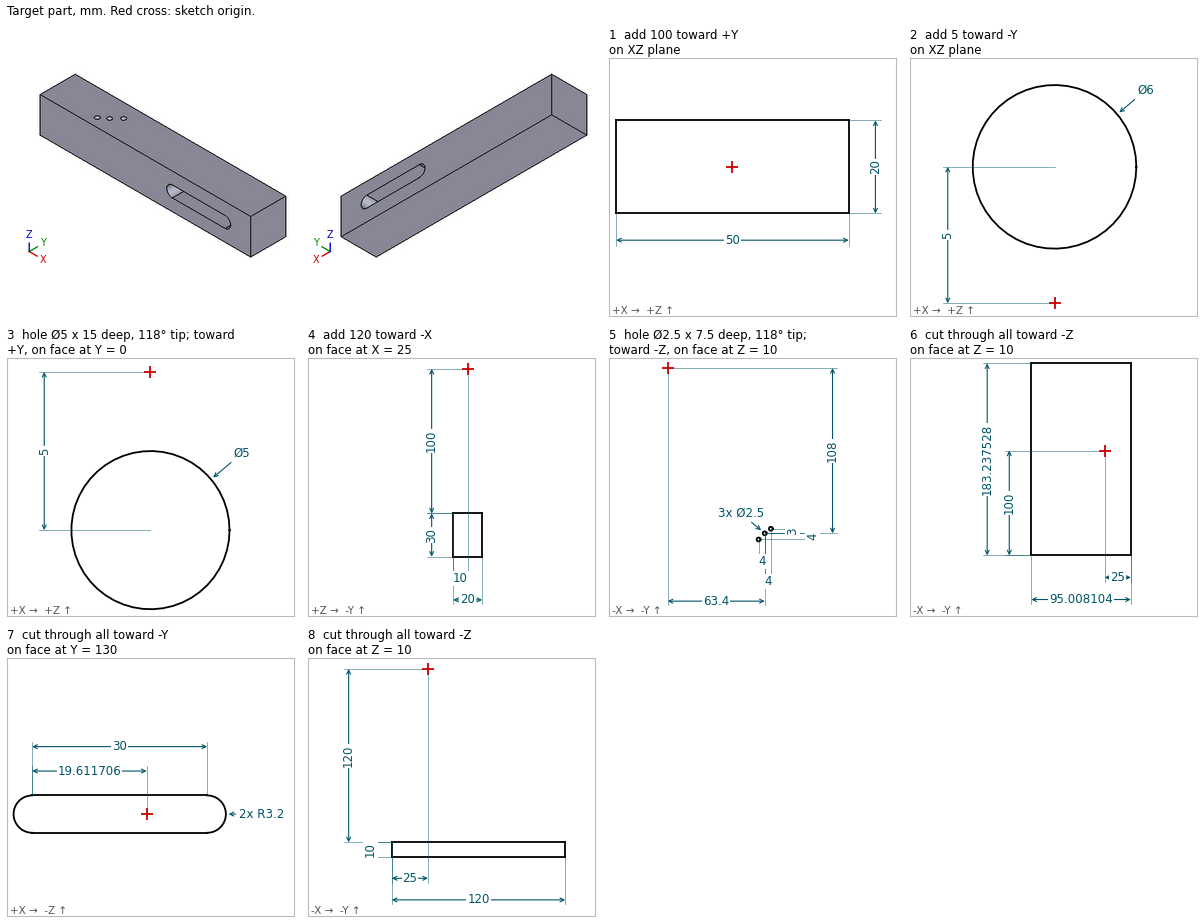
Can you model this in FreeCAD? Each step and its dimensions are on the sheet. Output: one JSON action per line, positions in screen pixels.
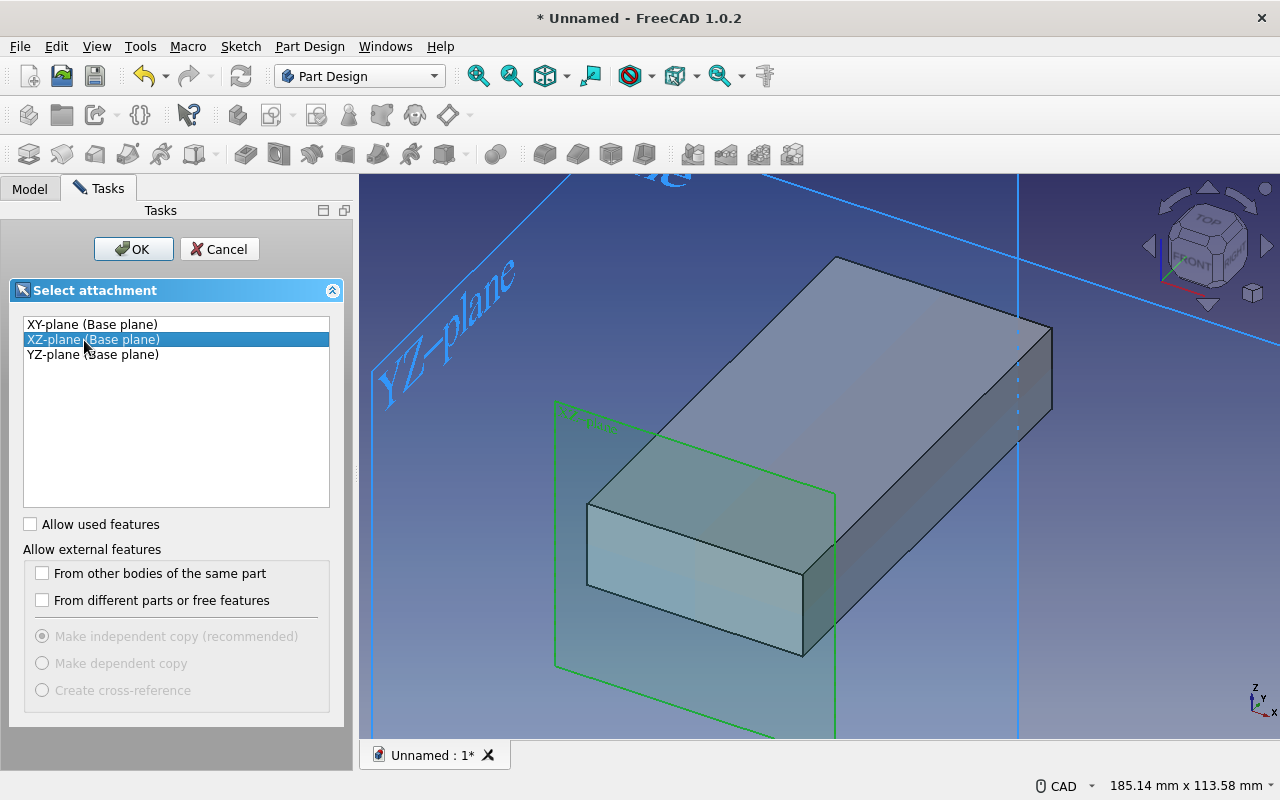
{"action": "left_click", "coordinate": [134, 249]}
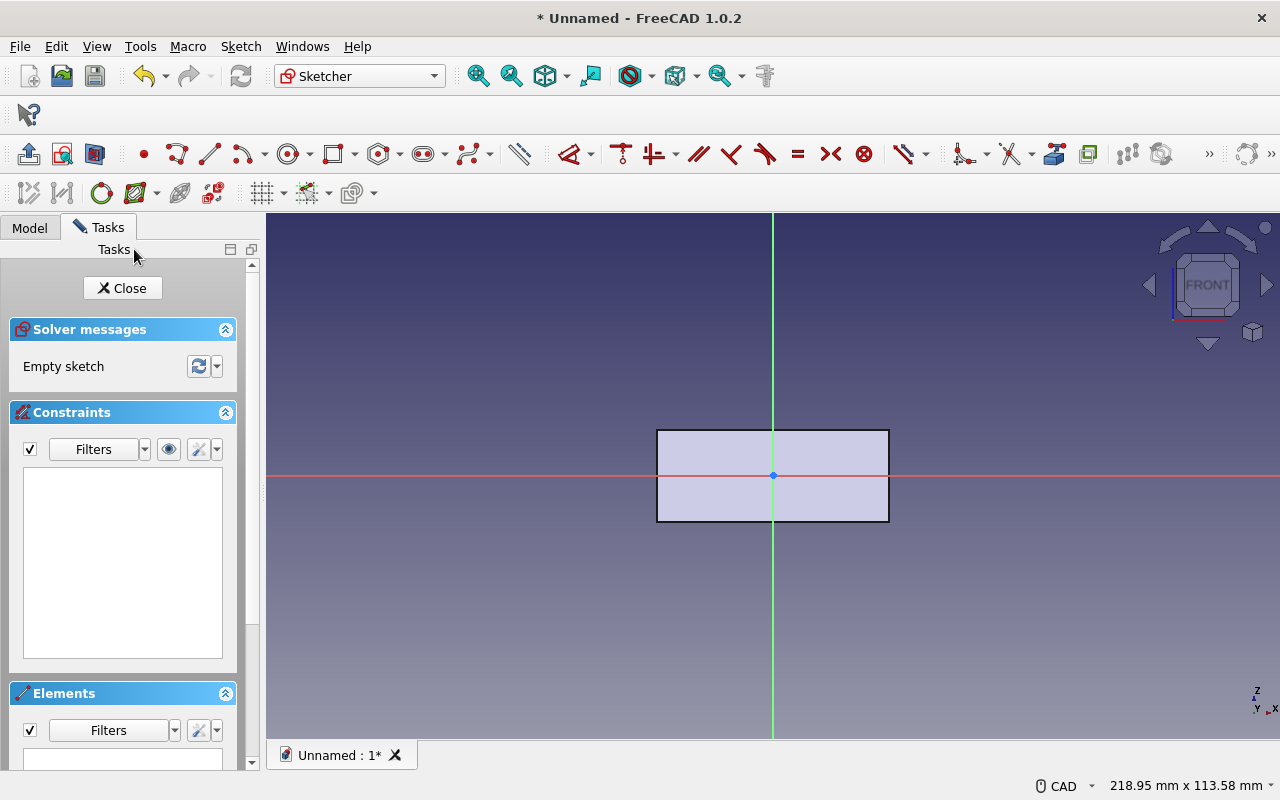
{"action": "scroll", "coordinate": [782, 455], "scroll_direction": "up", "scroll_amount": 11}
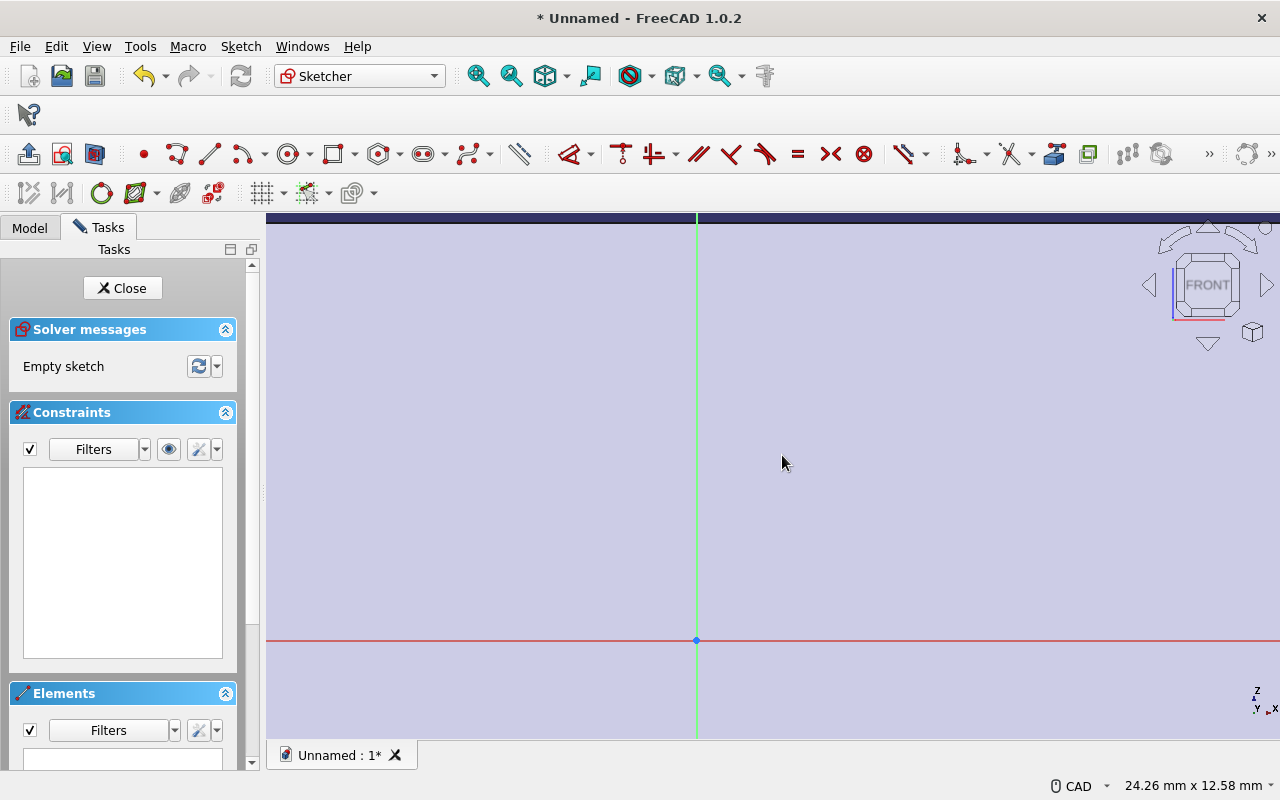
{"action": "left_click", "coordinate": [288, 154]}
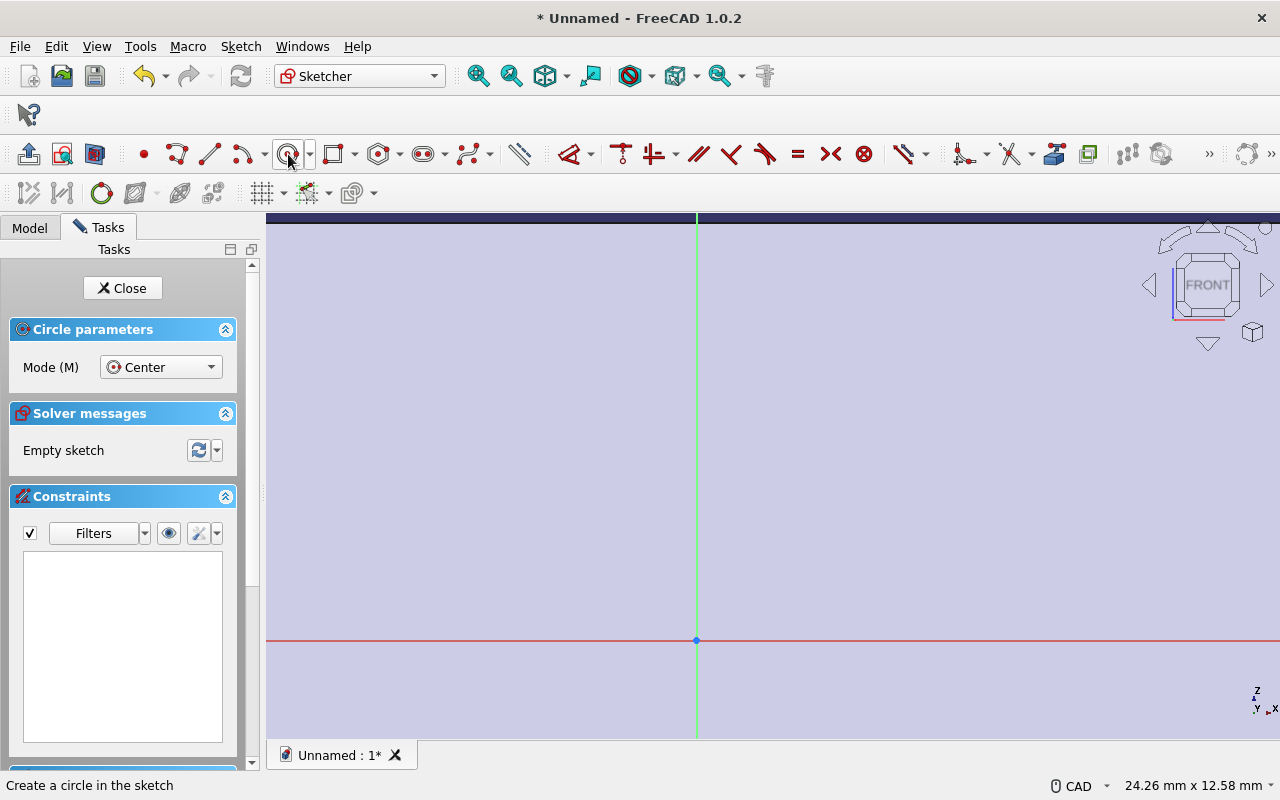
{"action": "left_click", "coordinate": [697, 432]}
{"action": "left_click", "coordinate": [785, 343]}
{"action": "key", "text": "Escape"}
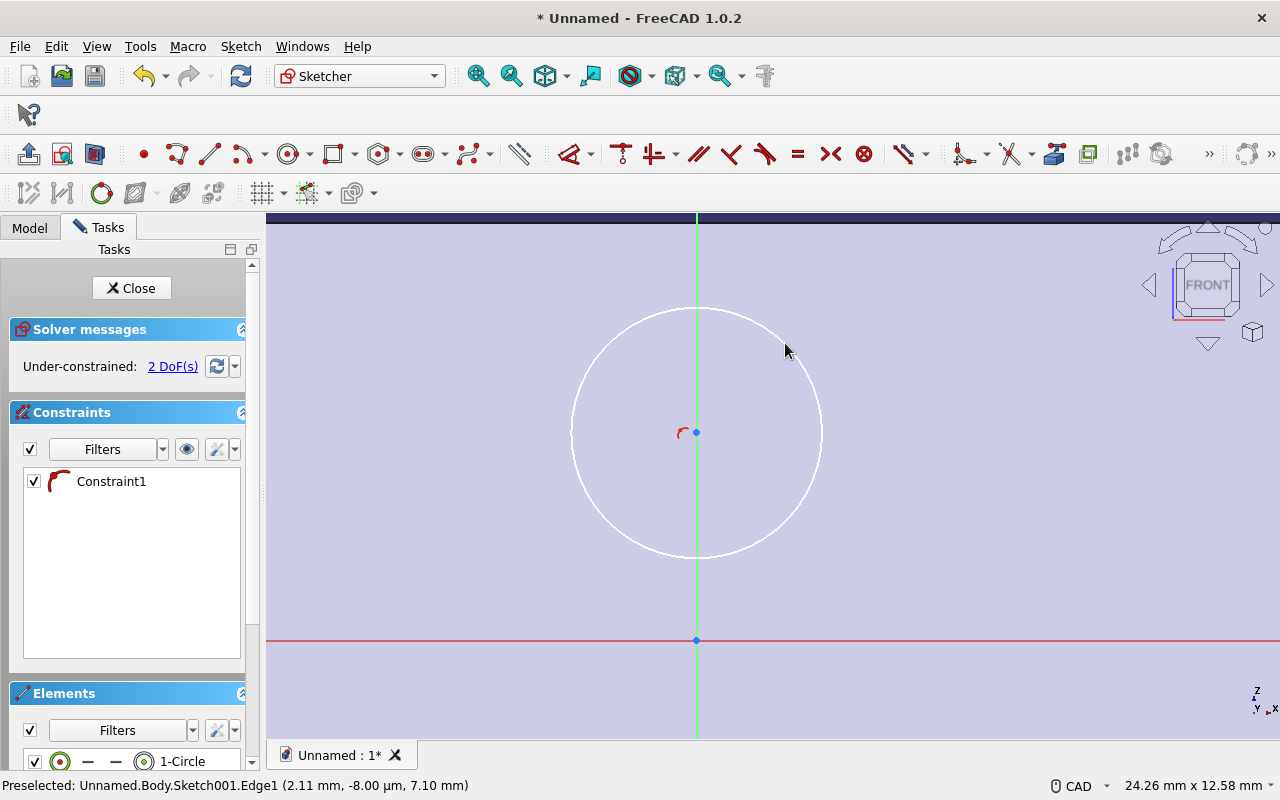
{"action": "left_click", "coordinate": [568, 154]}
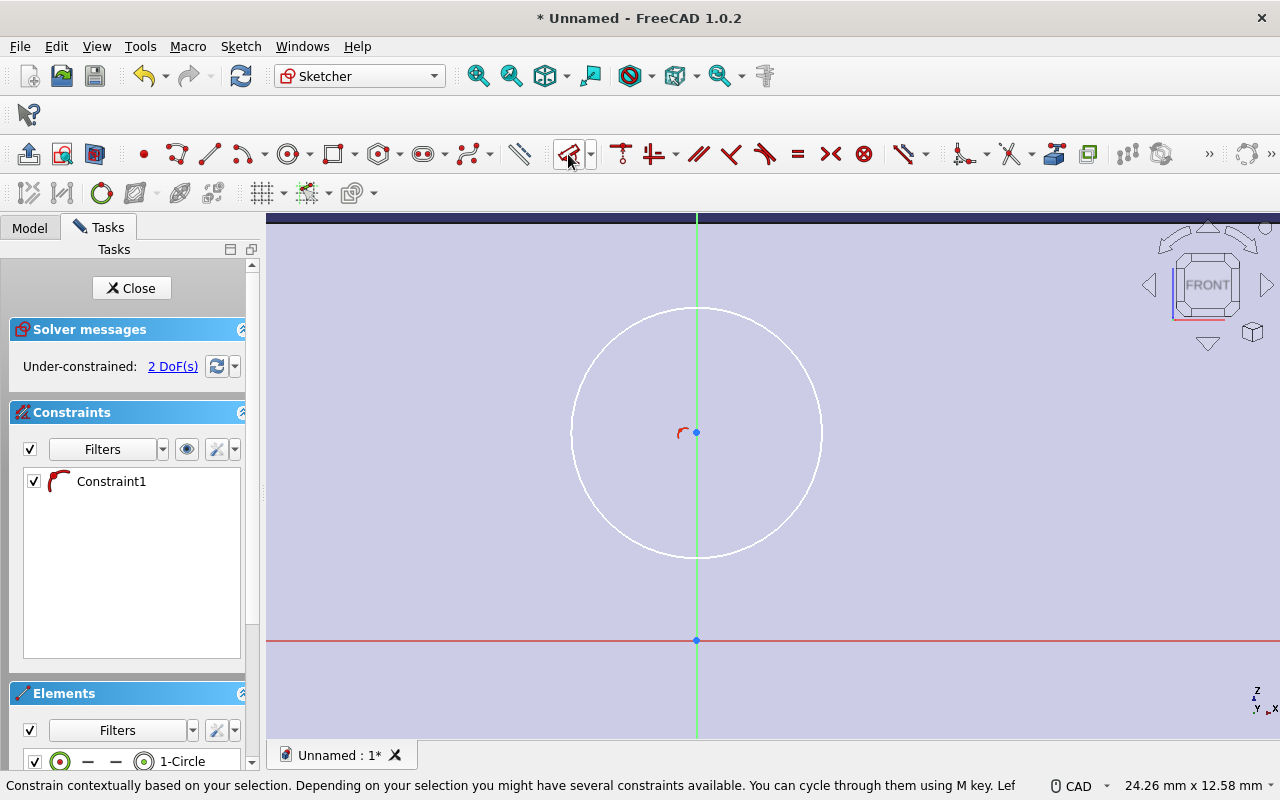
{"action": "left_click", "coordinate": [785, 344]}
{"action": "left_click", "coordinate": [808, 321]}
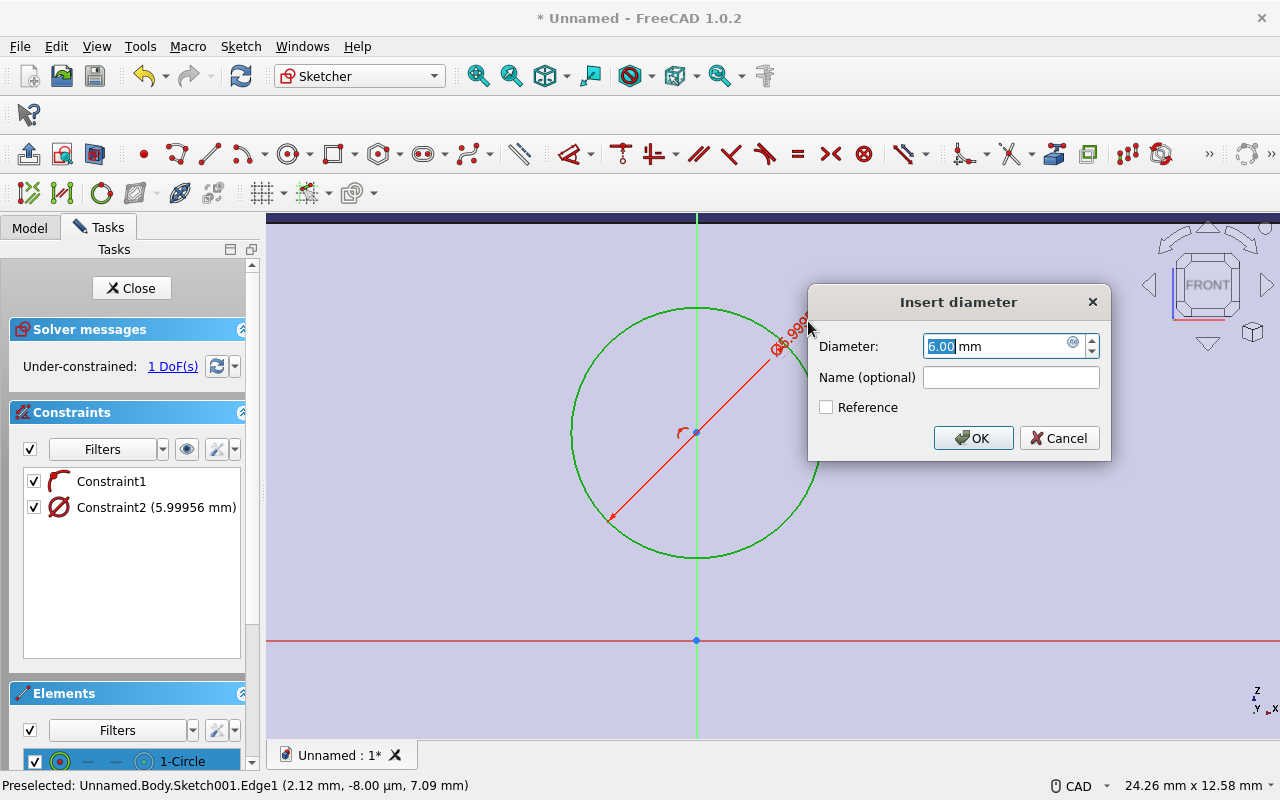
{"action": "type", "text": "6"}
{"action": "key", "text": "Return"}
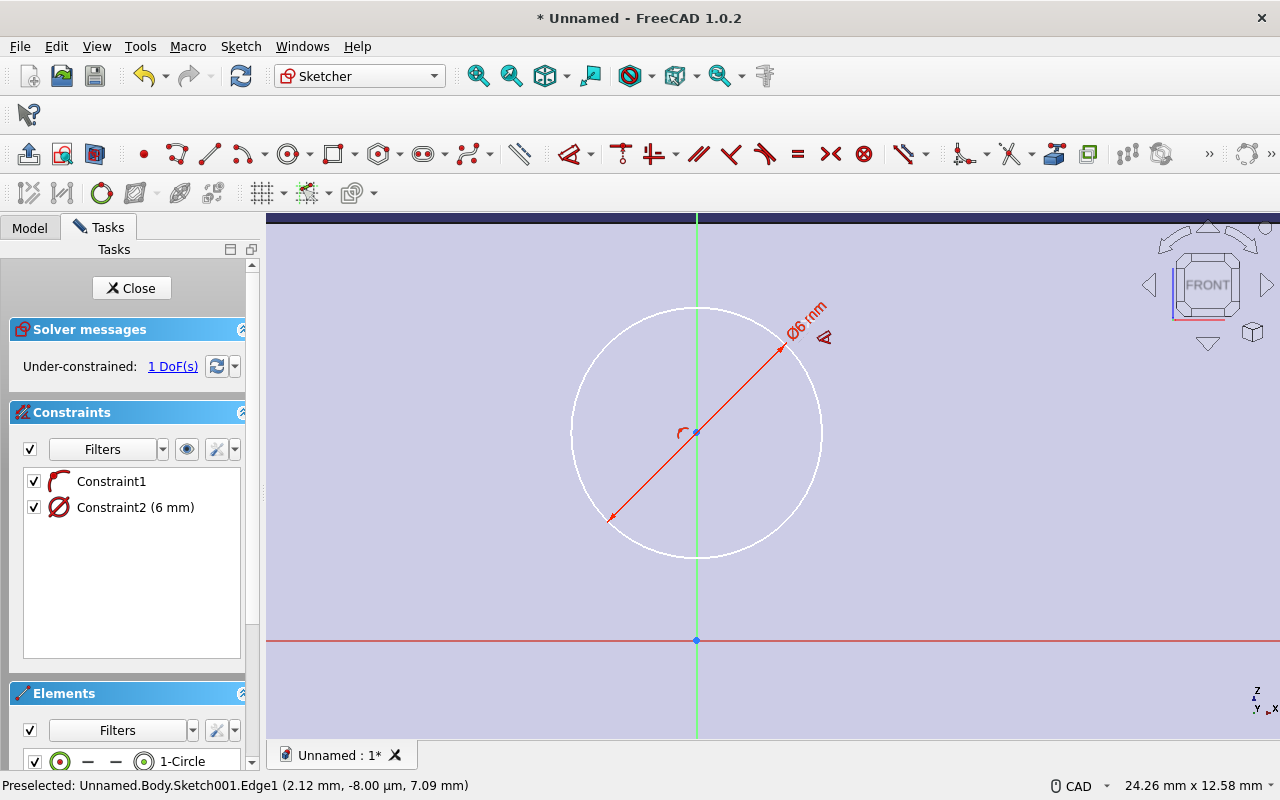
{"action": "left_click", "coordinate": [697, 433]}
{"action": "left_click", "coordinate": [731, 537]}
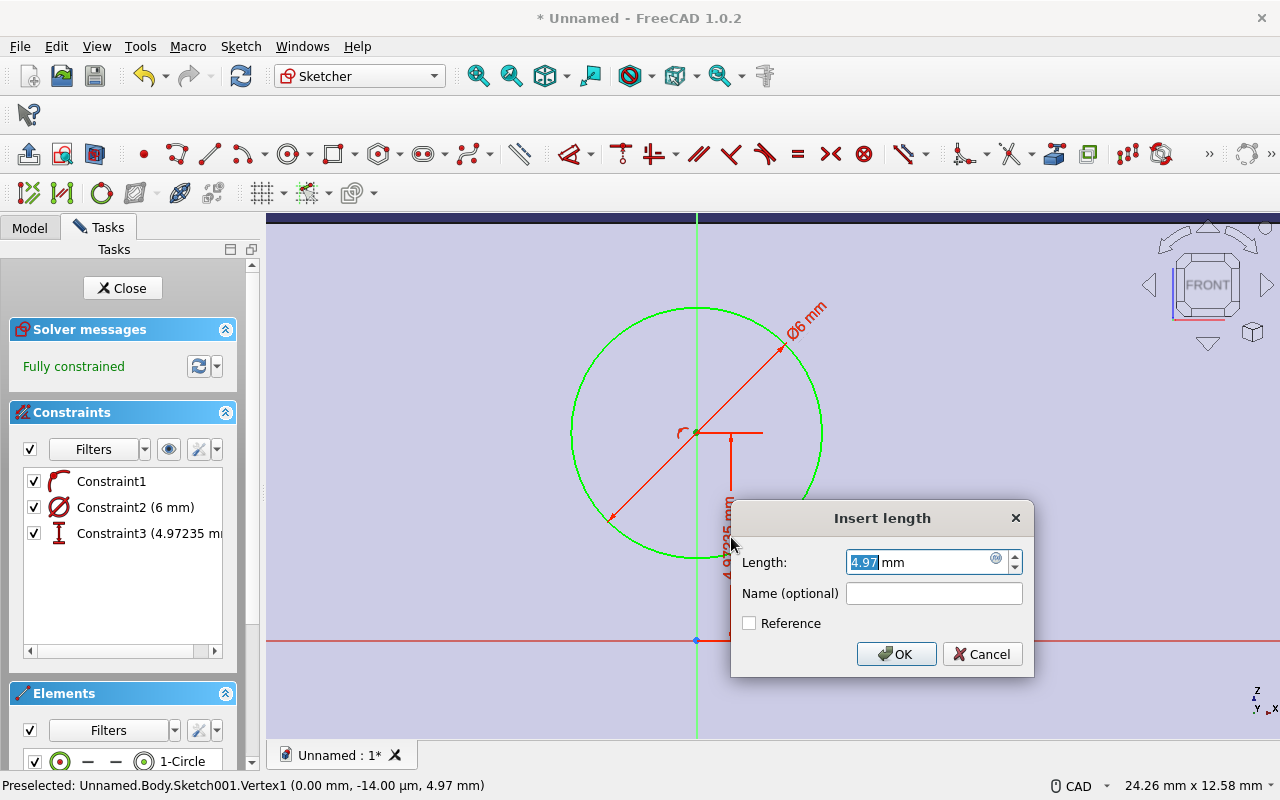
{"action": "type", "text": "5"}
{"action": "key", "text": "Return"}
{"action": "key", "text": "Escape"}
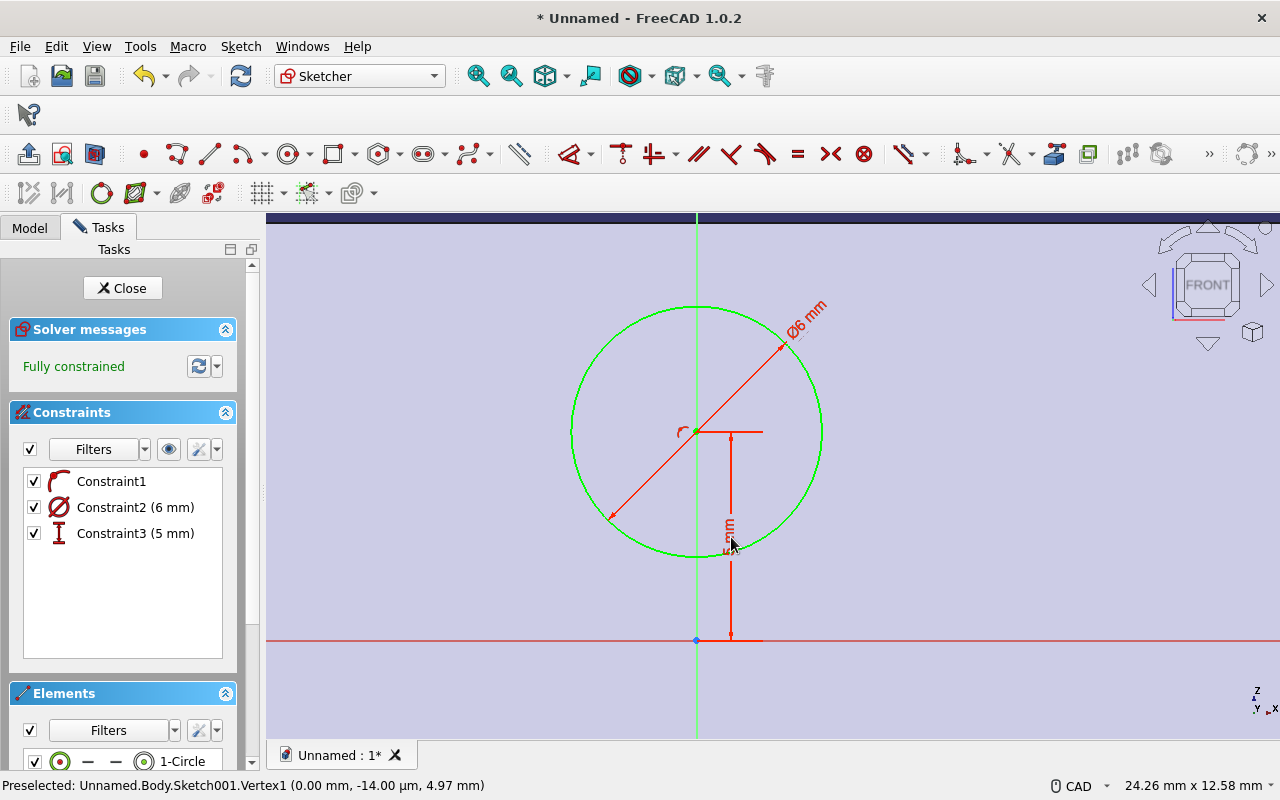
{"action": "left_click", "coordinate": [123, 288]}